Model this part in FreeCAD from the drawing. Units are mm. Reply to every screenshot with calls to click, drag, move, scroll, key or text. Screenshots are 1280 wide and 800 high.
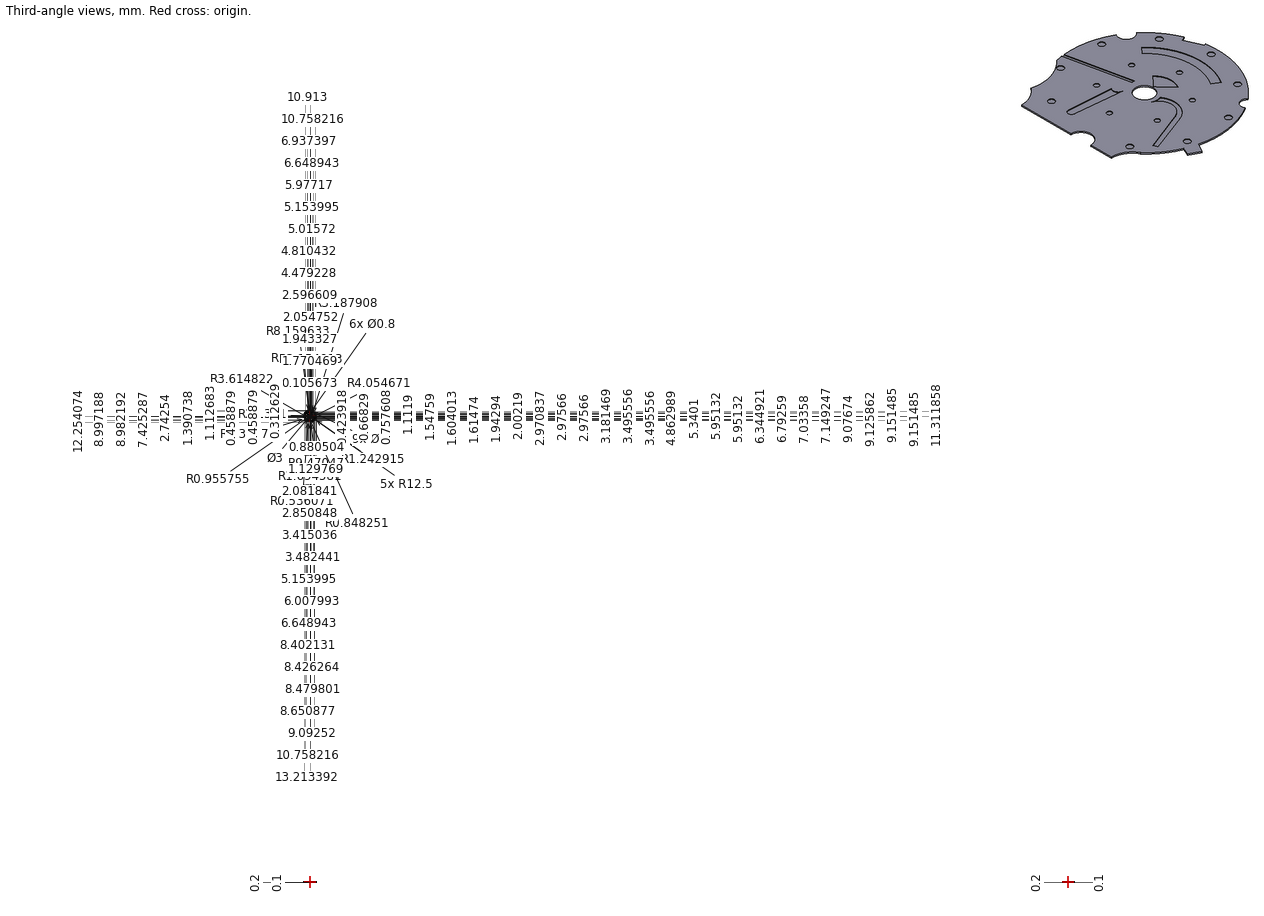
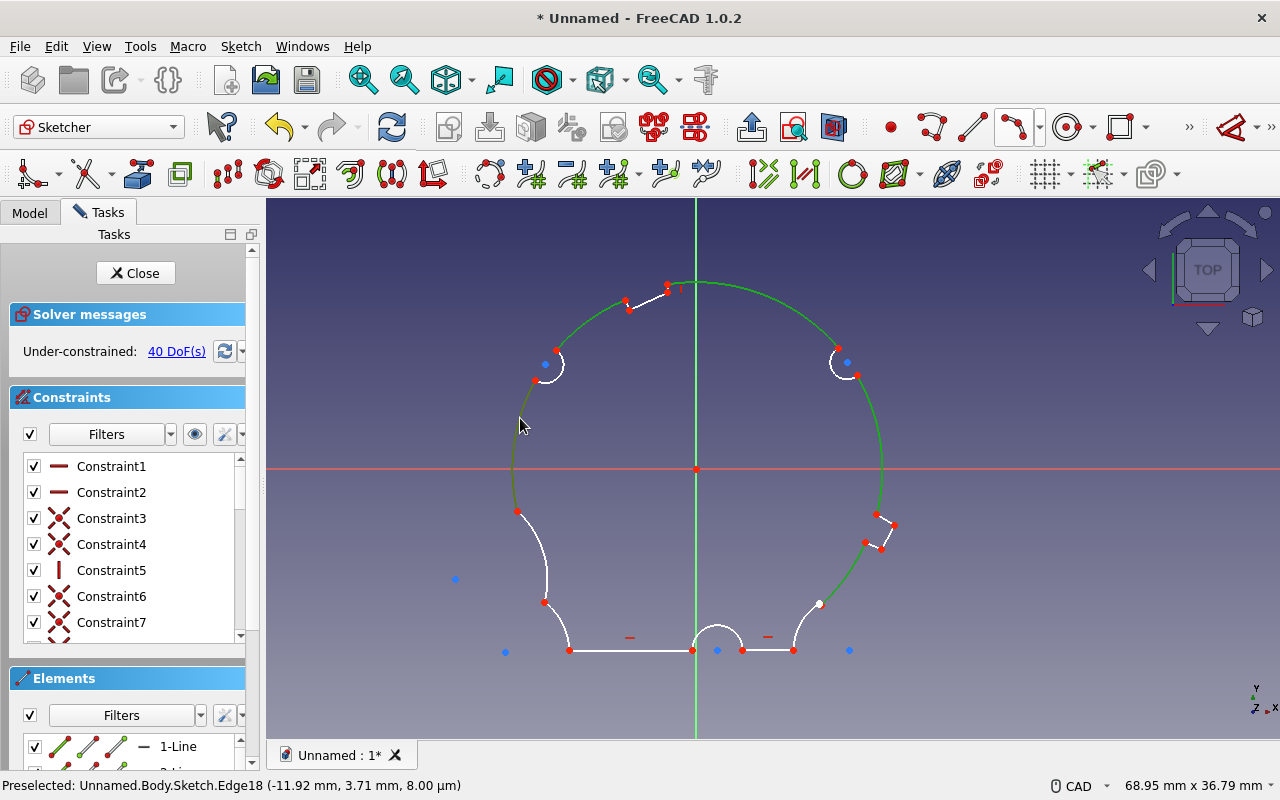
key(e)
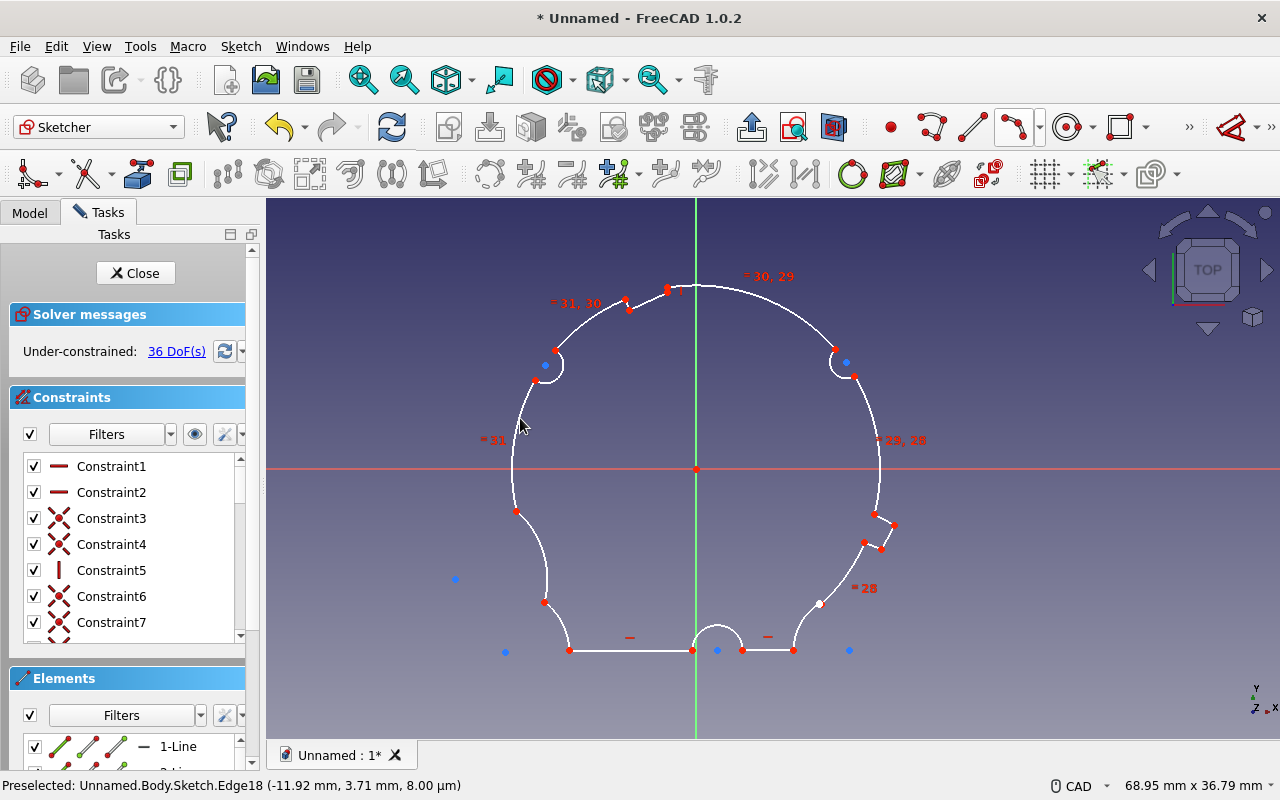
key(d)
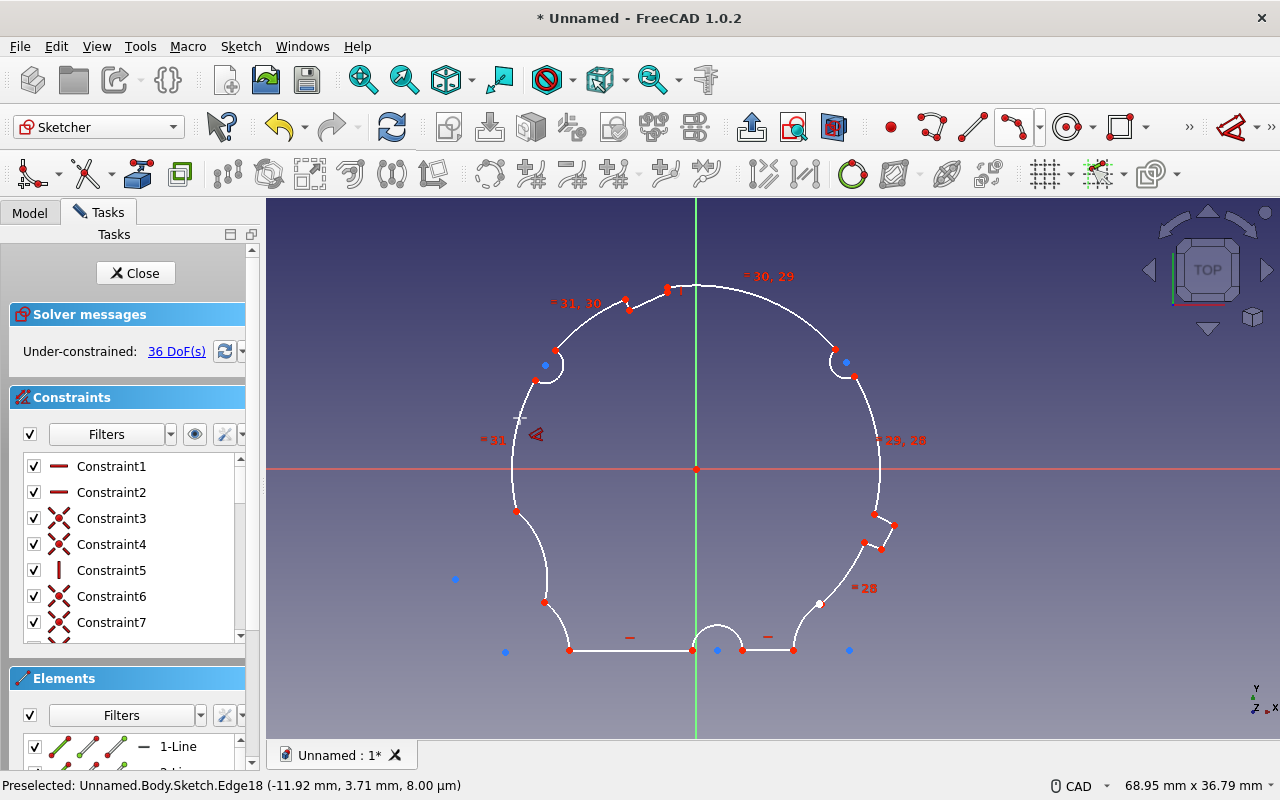
scroll(732, 630, up, 3)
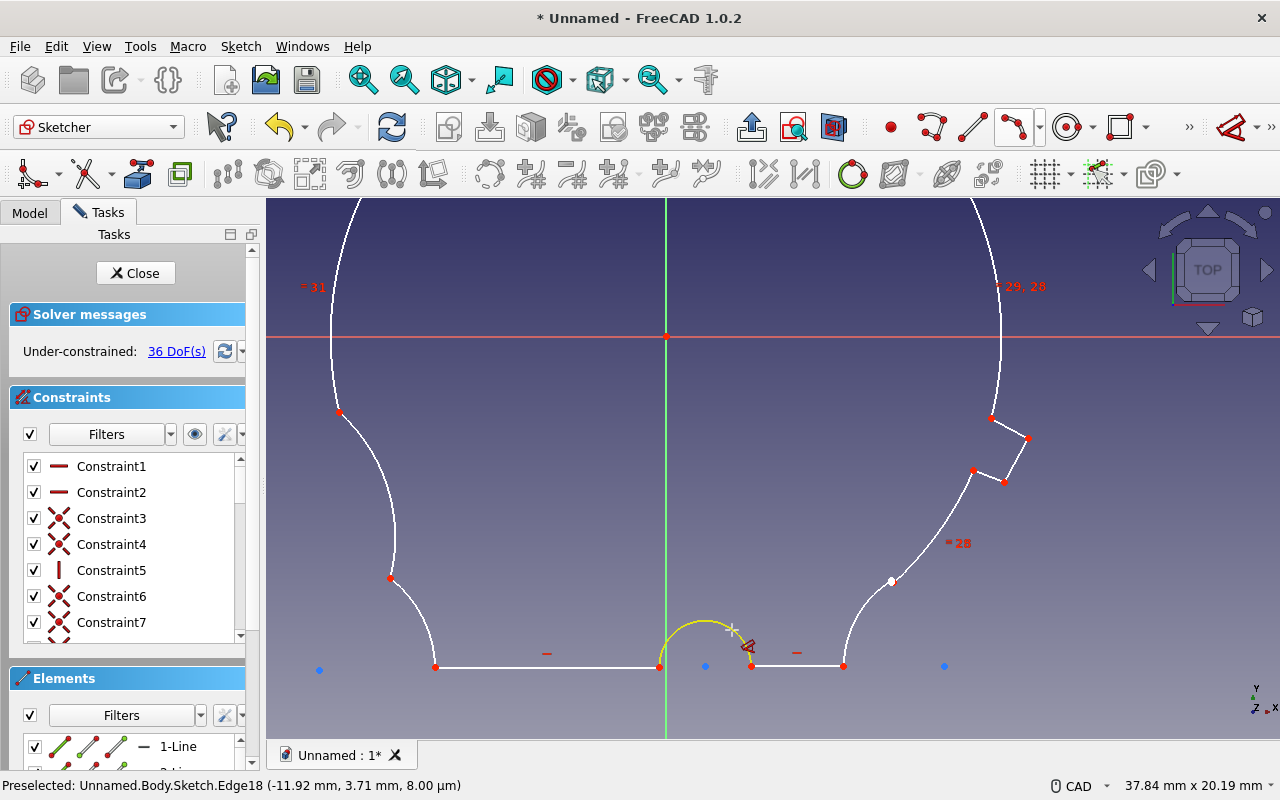
click(732, 629)
click(751, 603)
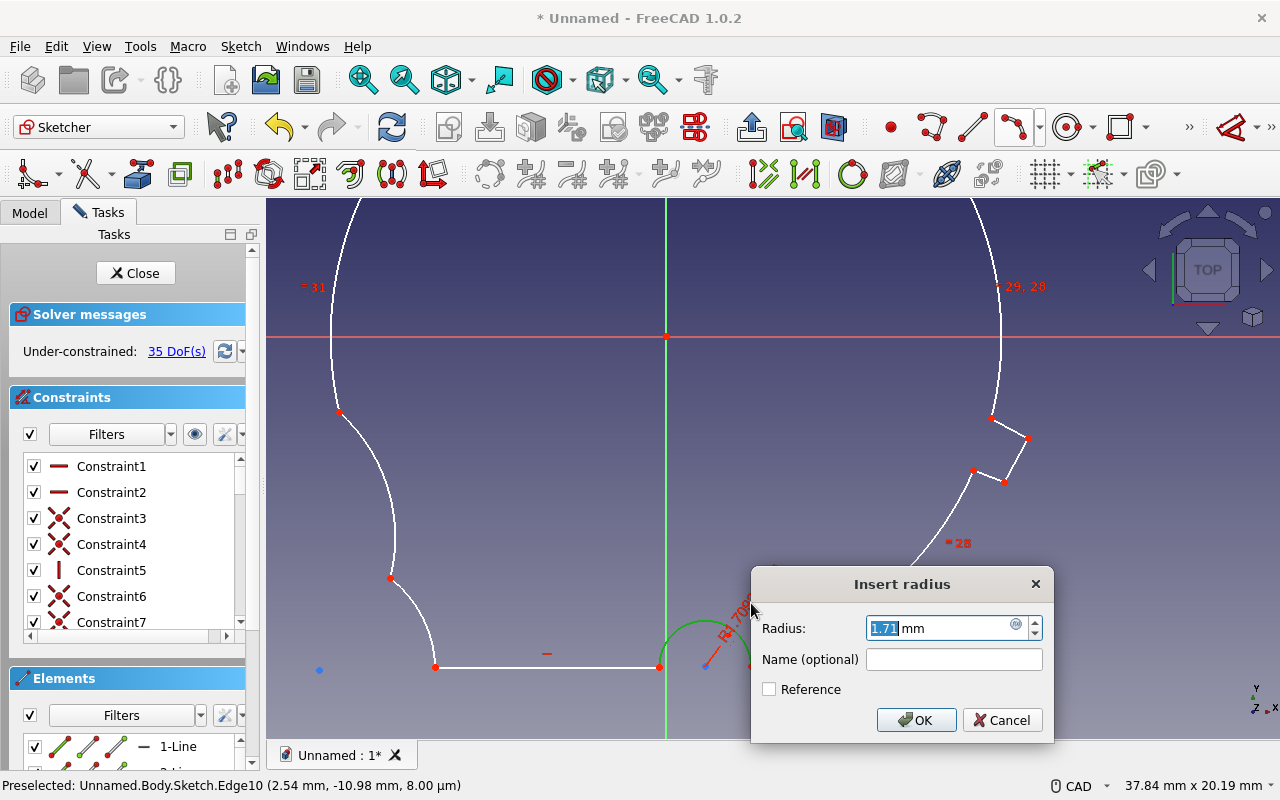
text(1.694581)
key(Return)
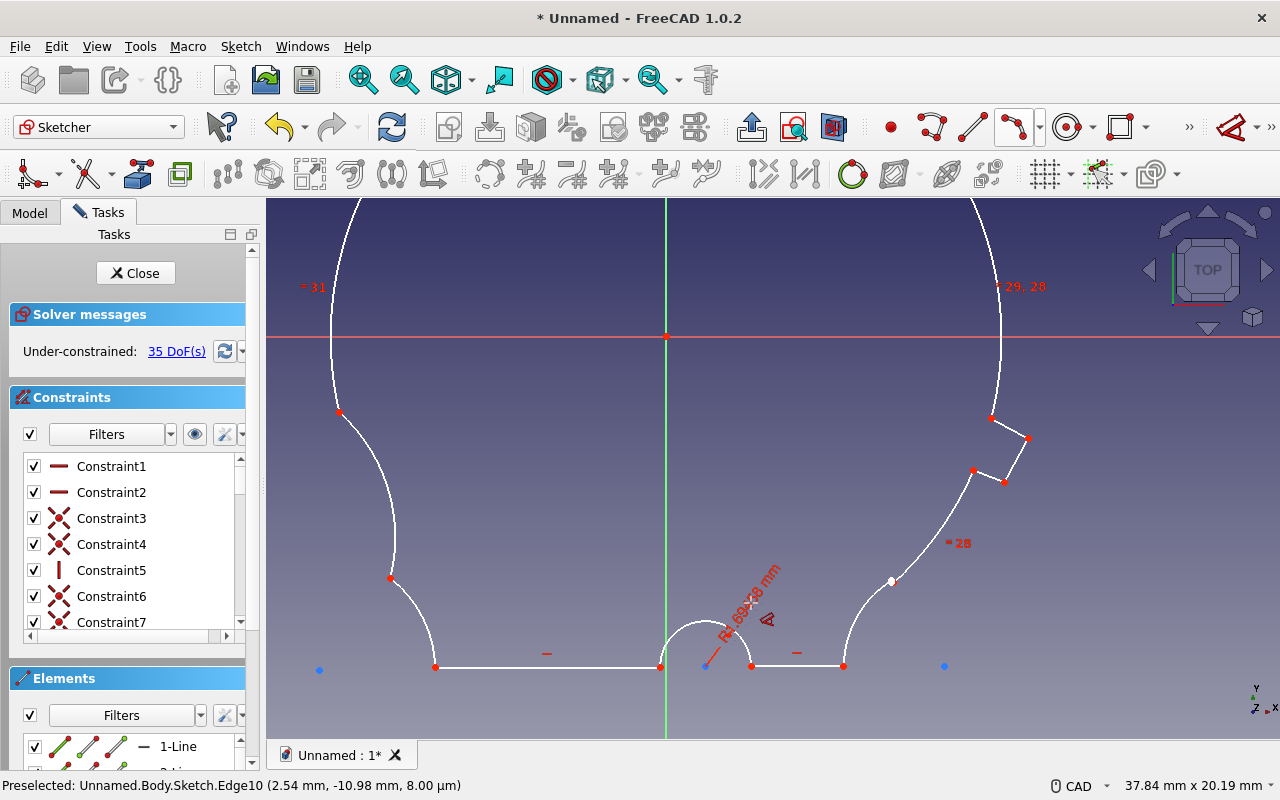
click(868, 601)
click(844, 580)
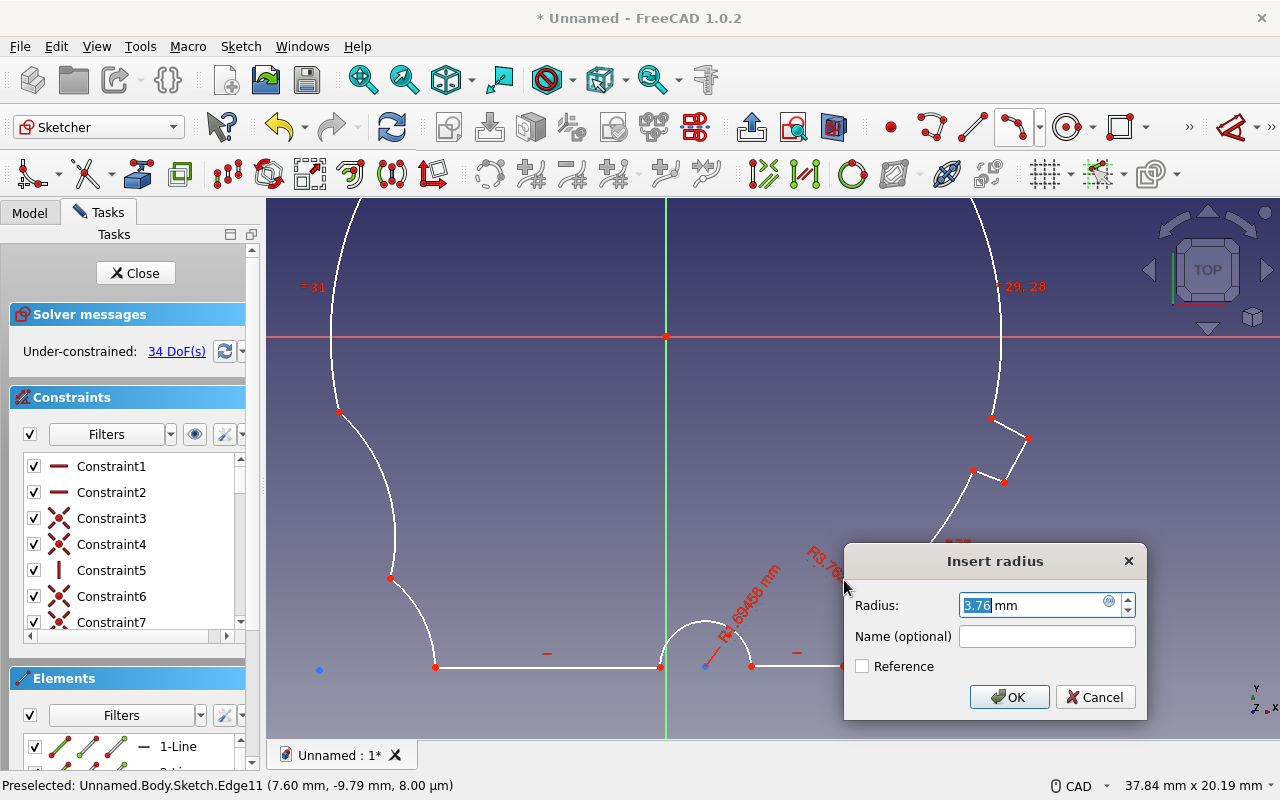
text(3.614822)
key(Return)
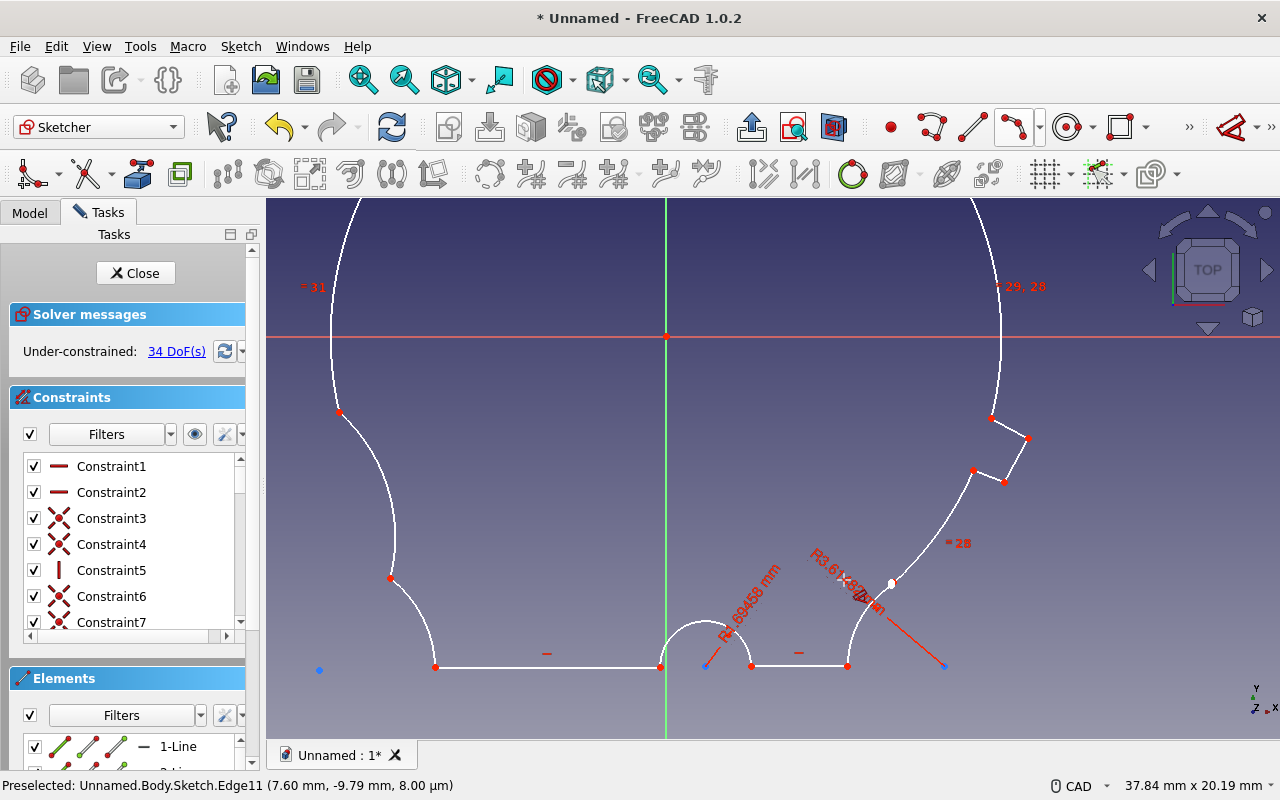
click(923, 553)
click(947, 574)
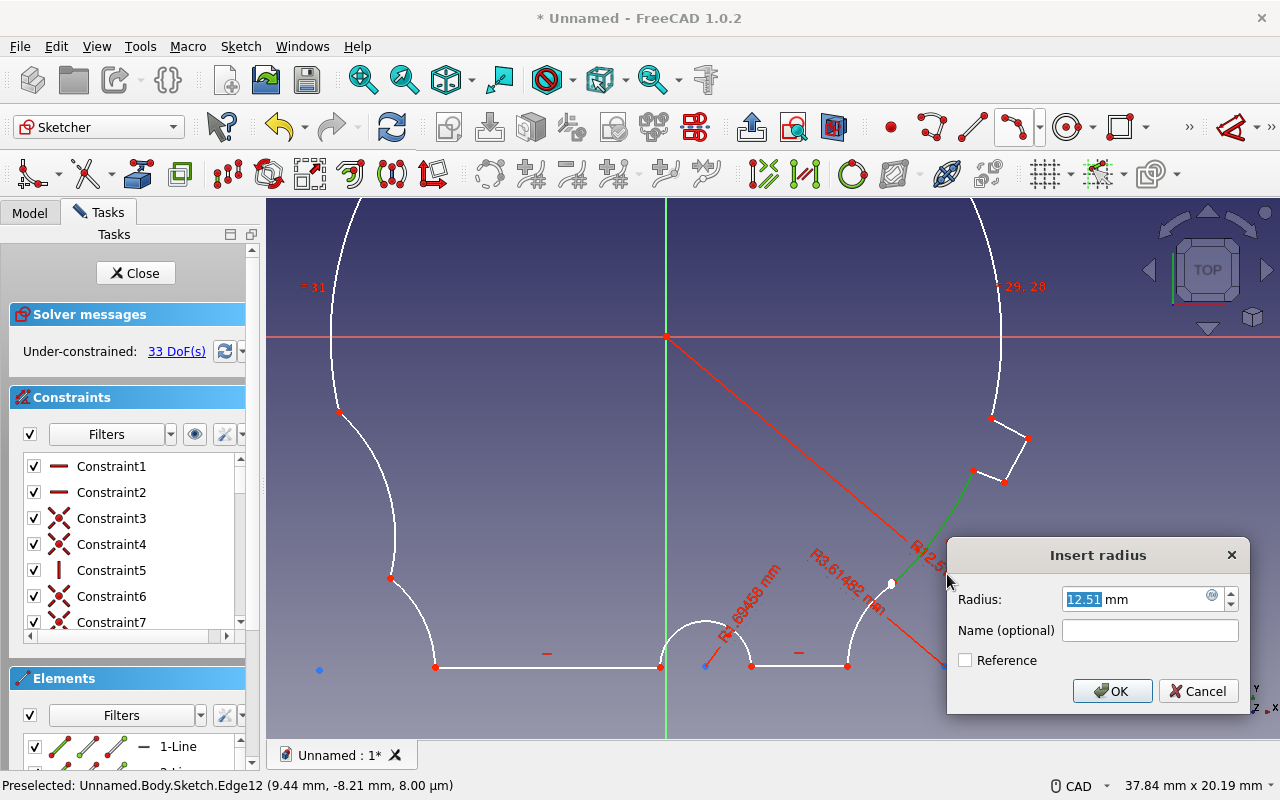
text(12.5)
key(Return)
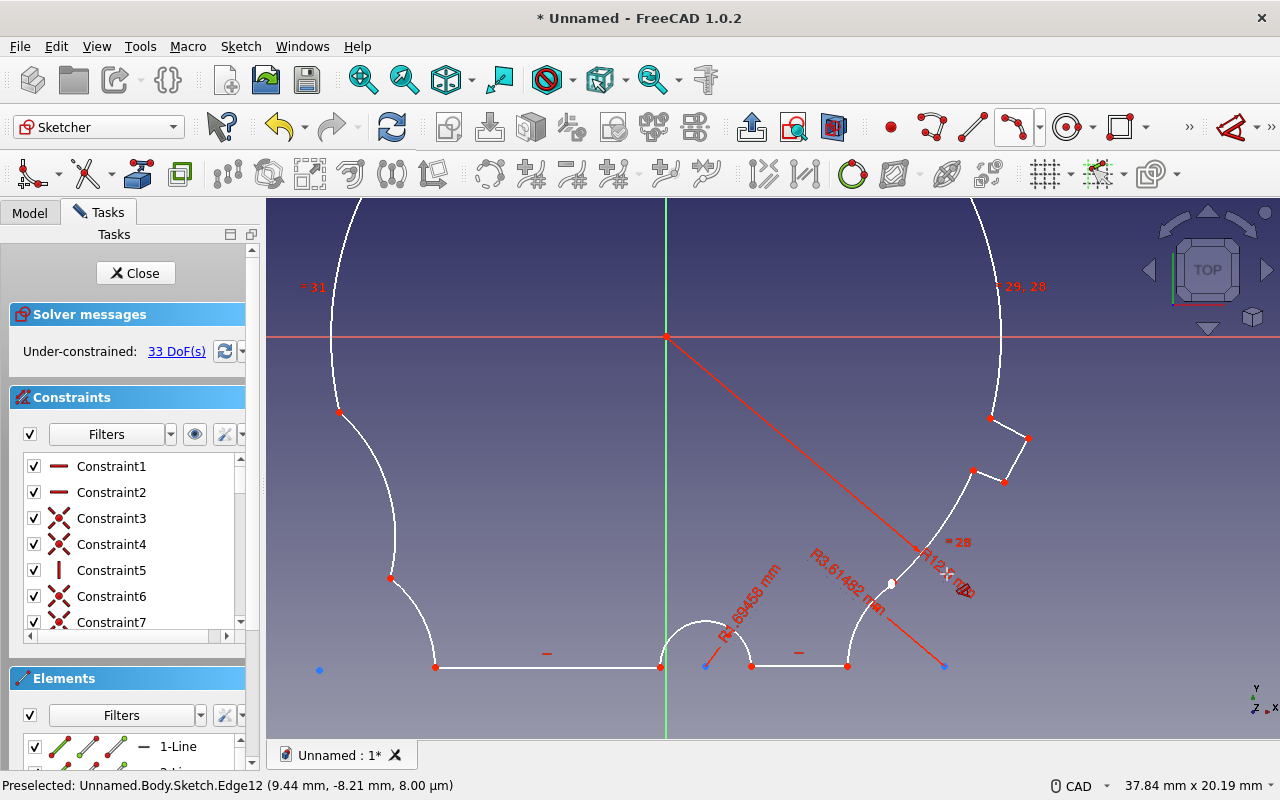
scroll(732, 630, down, 3)